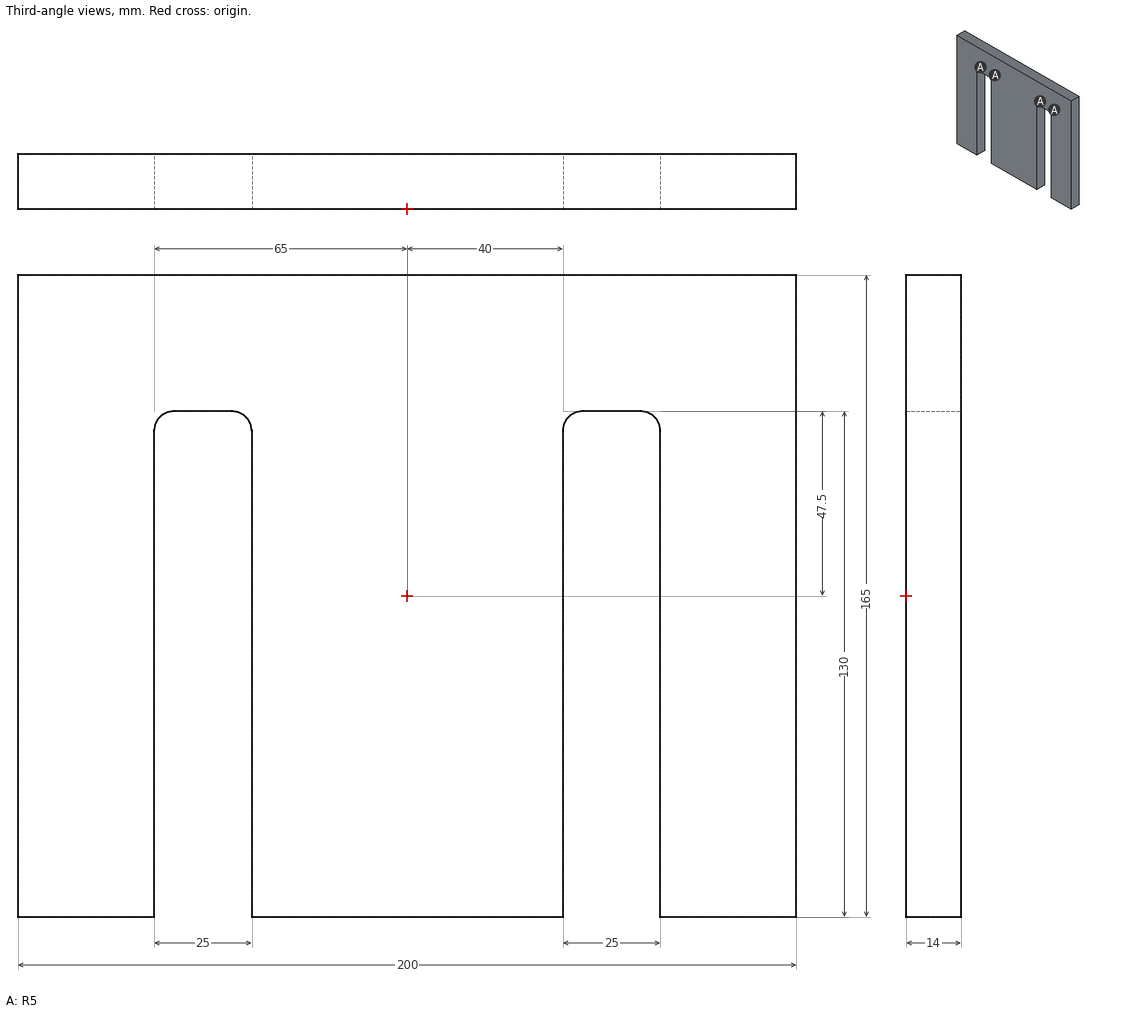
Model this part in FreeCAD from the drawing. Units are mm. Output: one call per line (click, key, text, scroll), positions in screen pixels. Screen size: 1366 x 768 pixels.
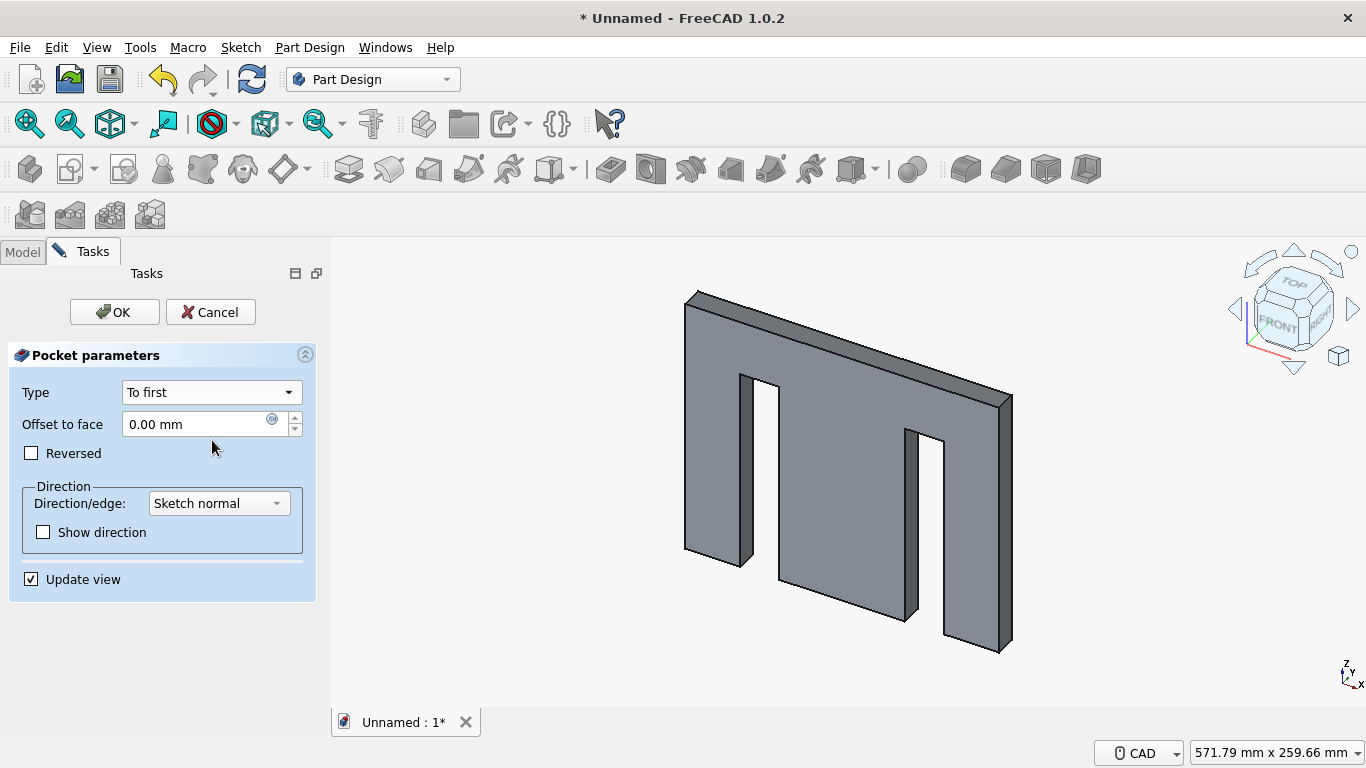
click(115, 312)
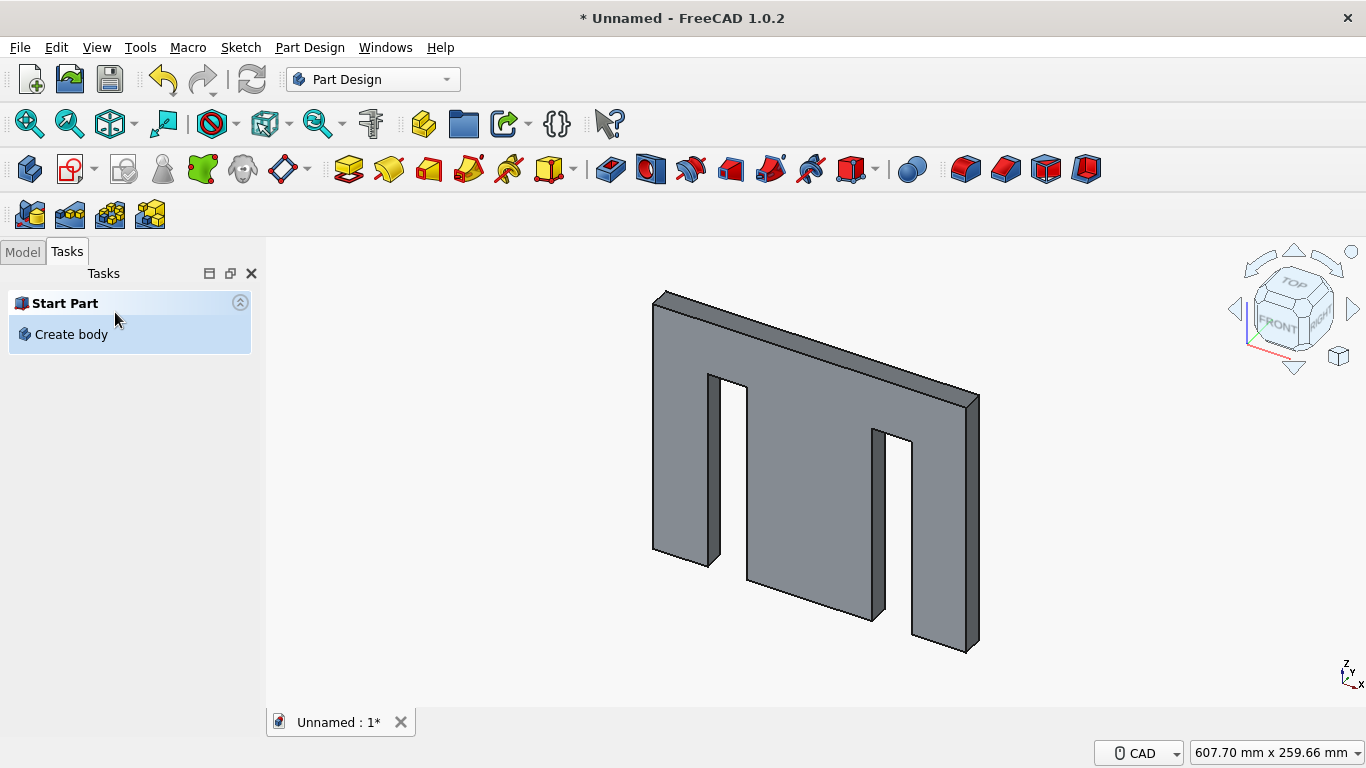
key(0)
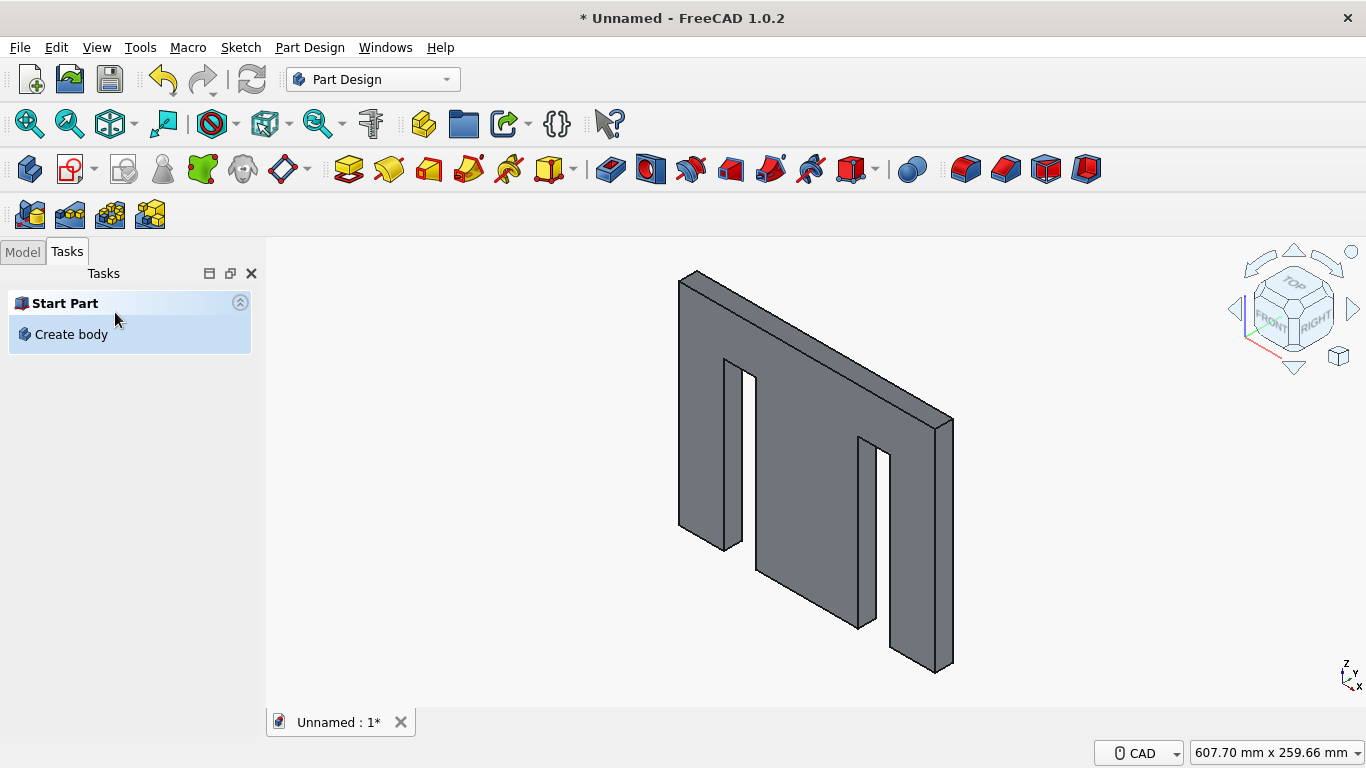
key(2)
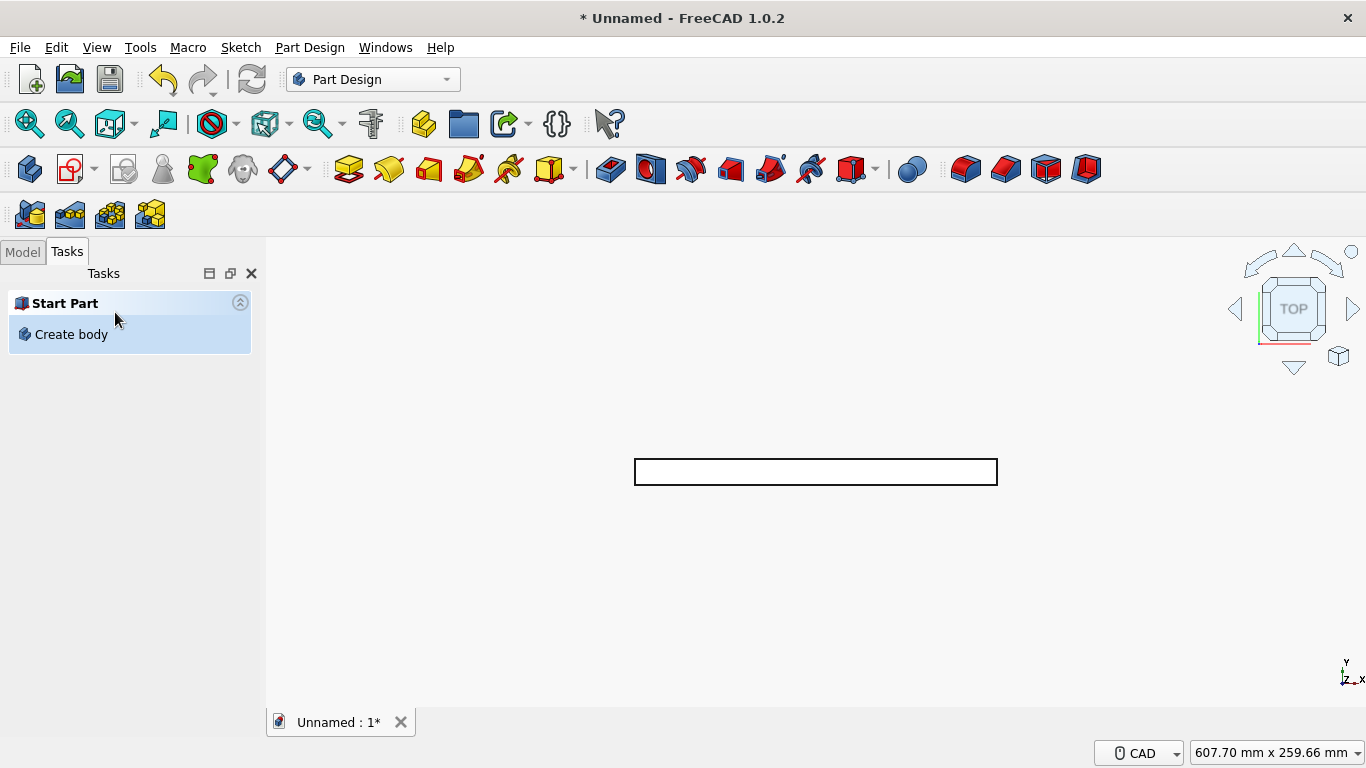
click(30, 124)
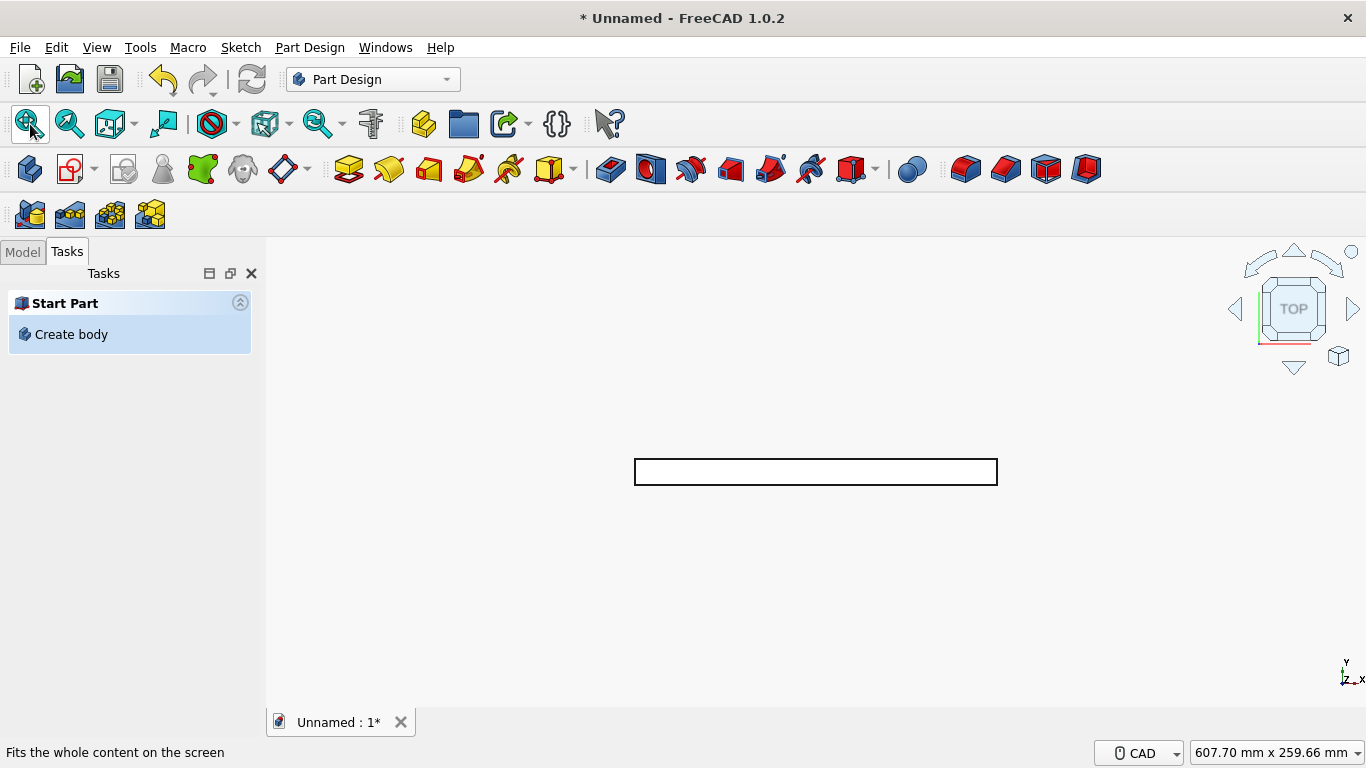
key(1)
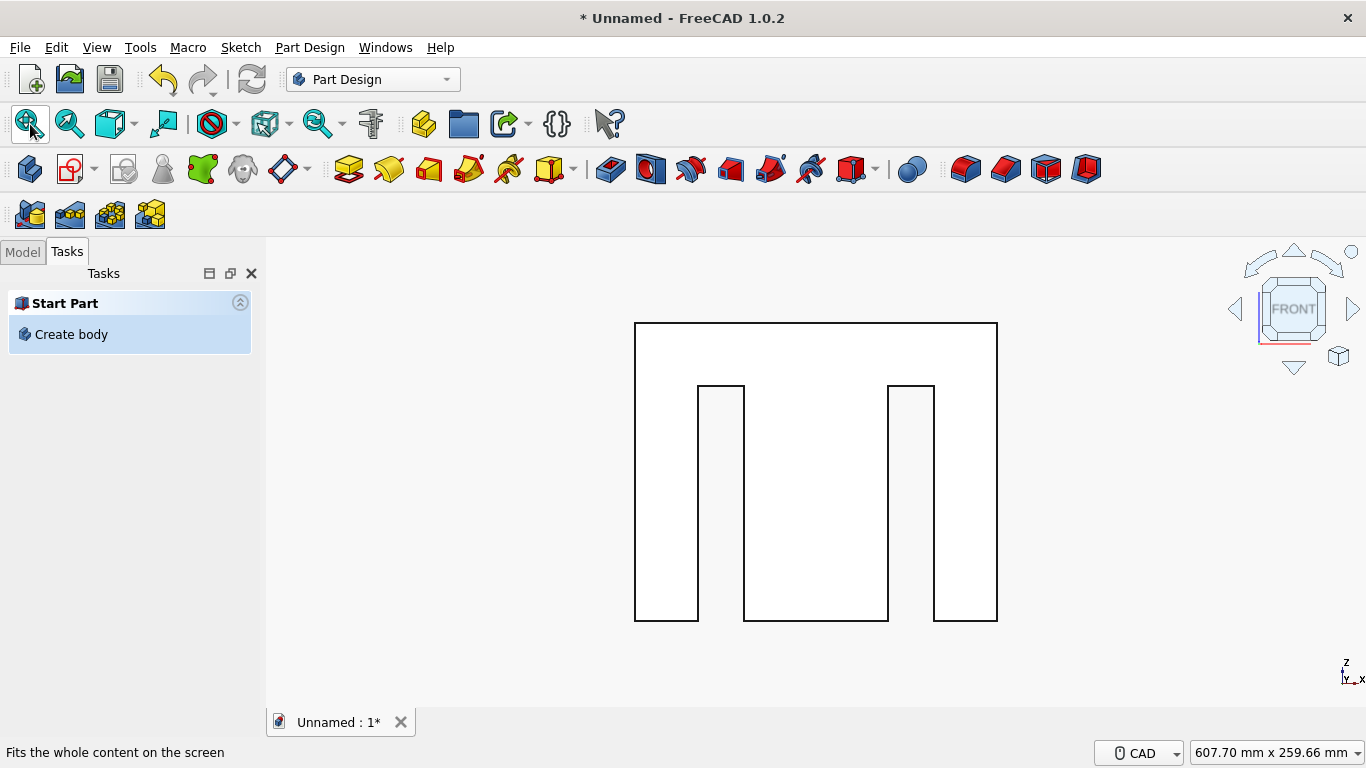
key(3)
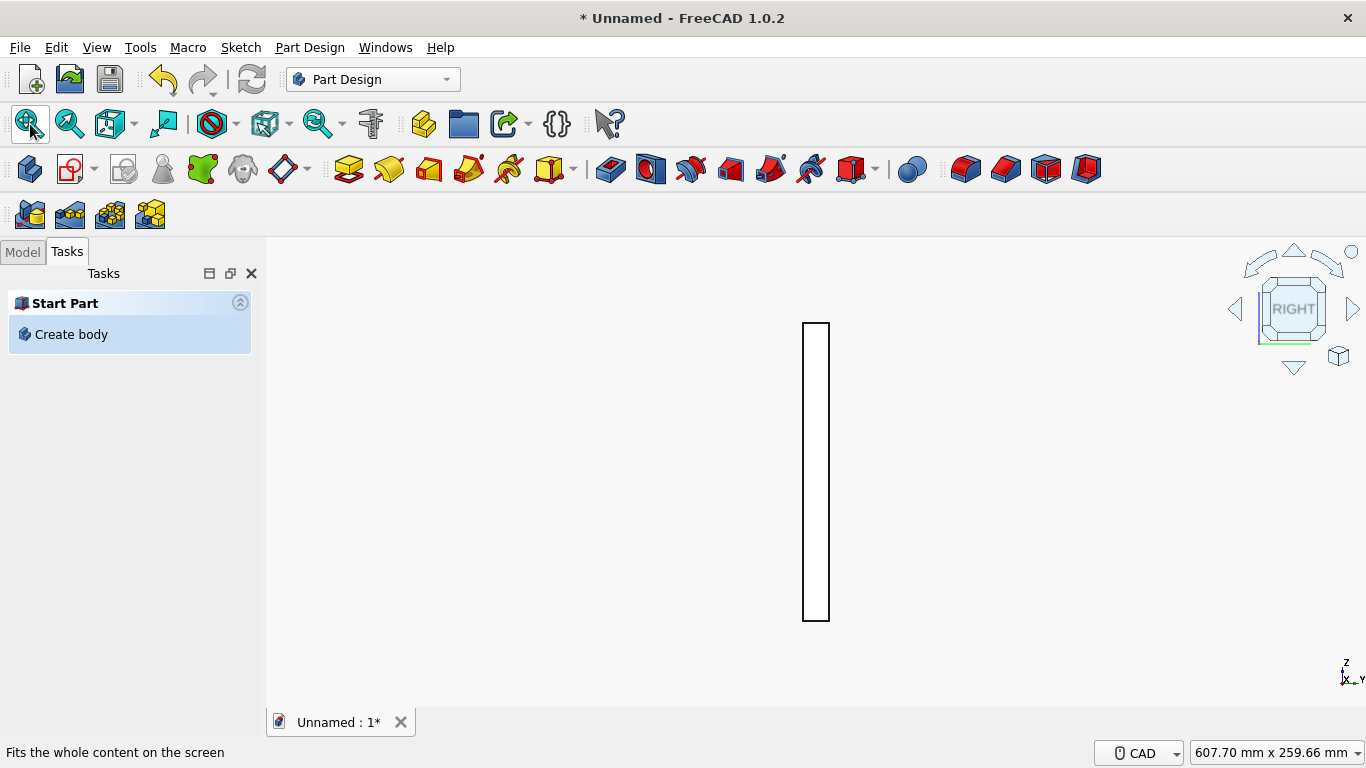
key(5)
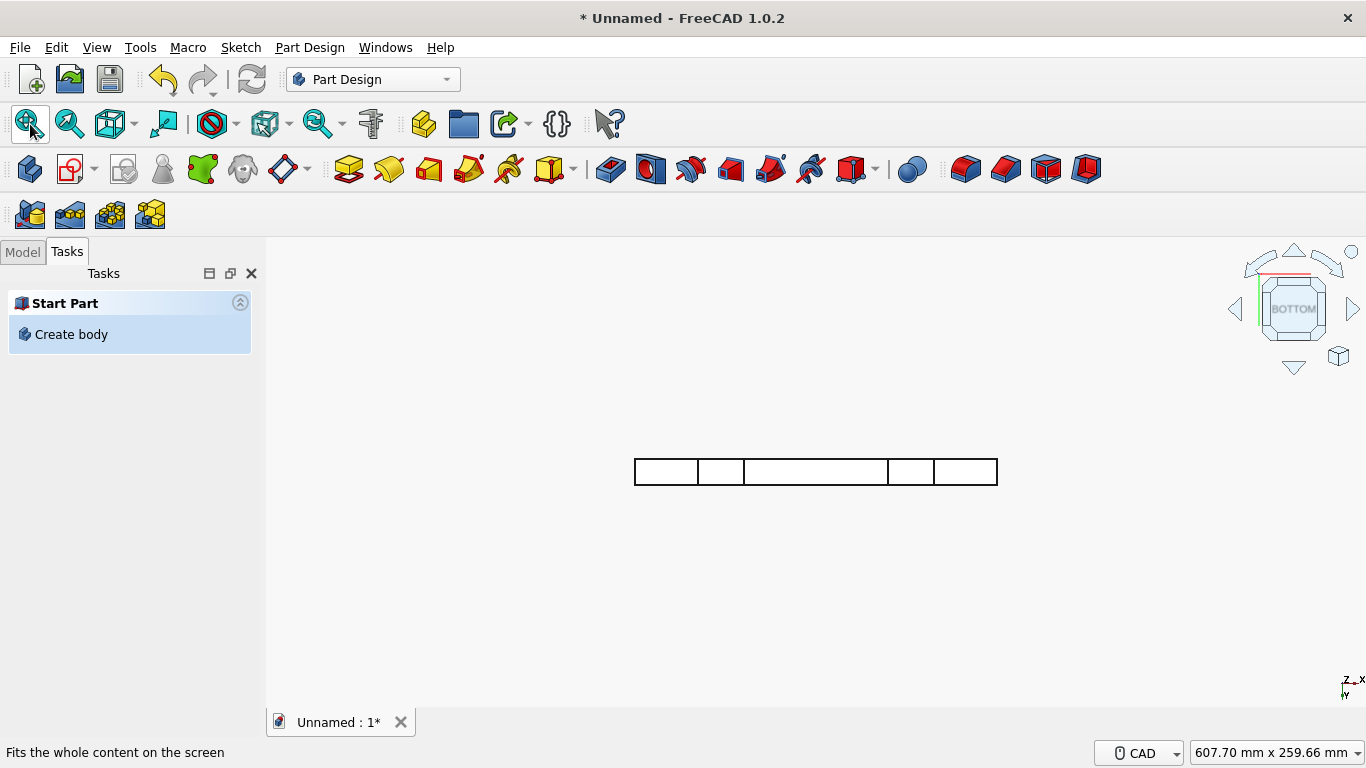
click(30, 124)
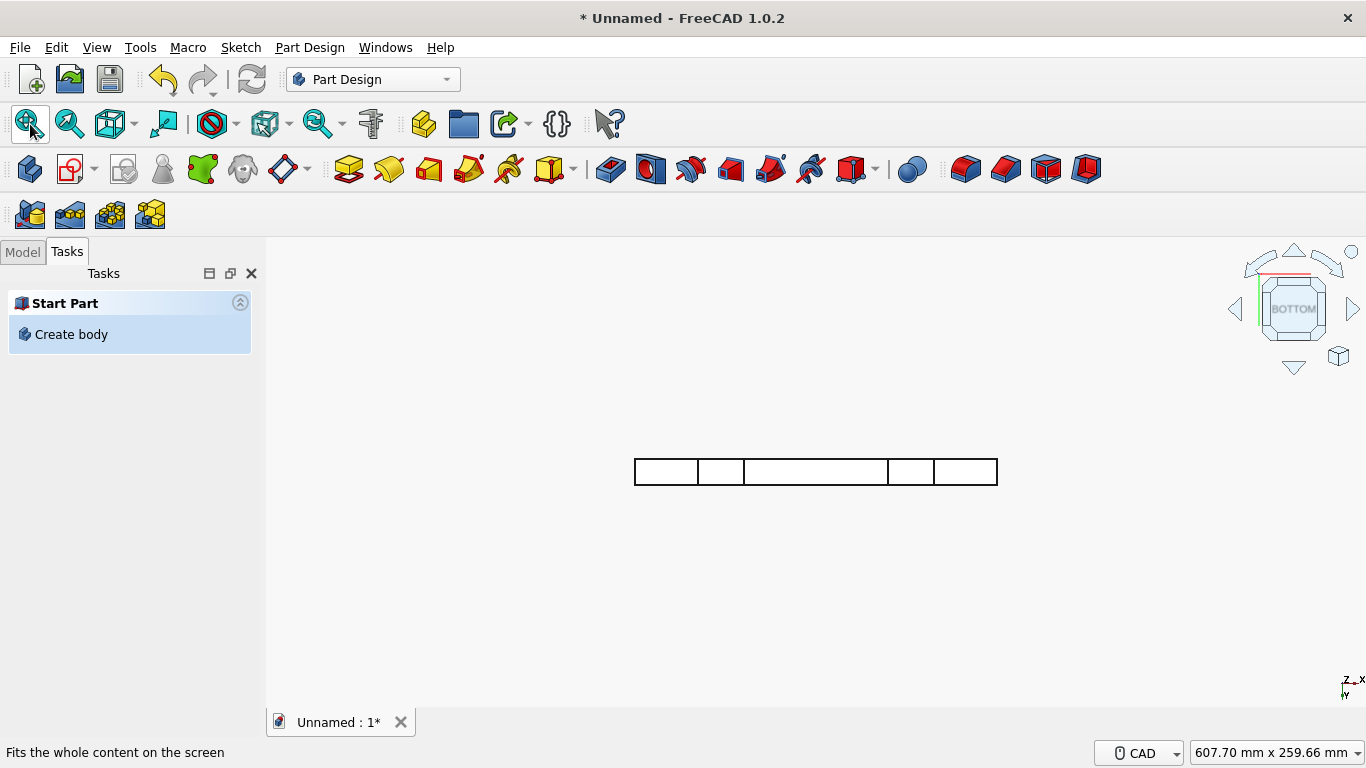
key(4)